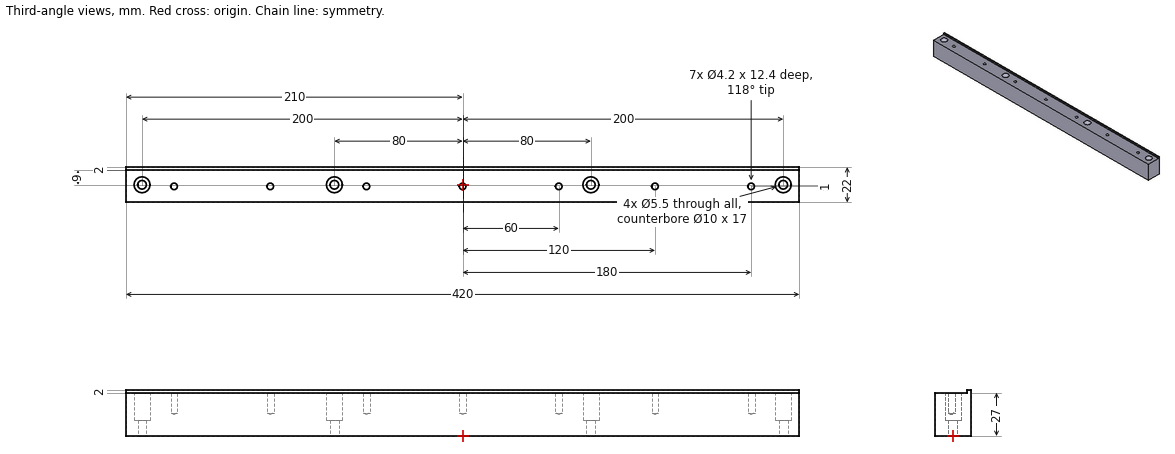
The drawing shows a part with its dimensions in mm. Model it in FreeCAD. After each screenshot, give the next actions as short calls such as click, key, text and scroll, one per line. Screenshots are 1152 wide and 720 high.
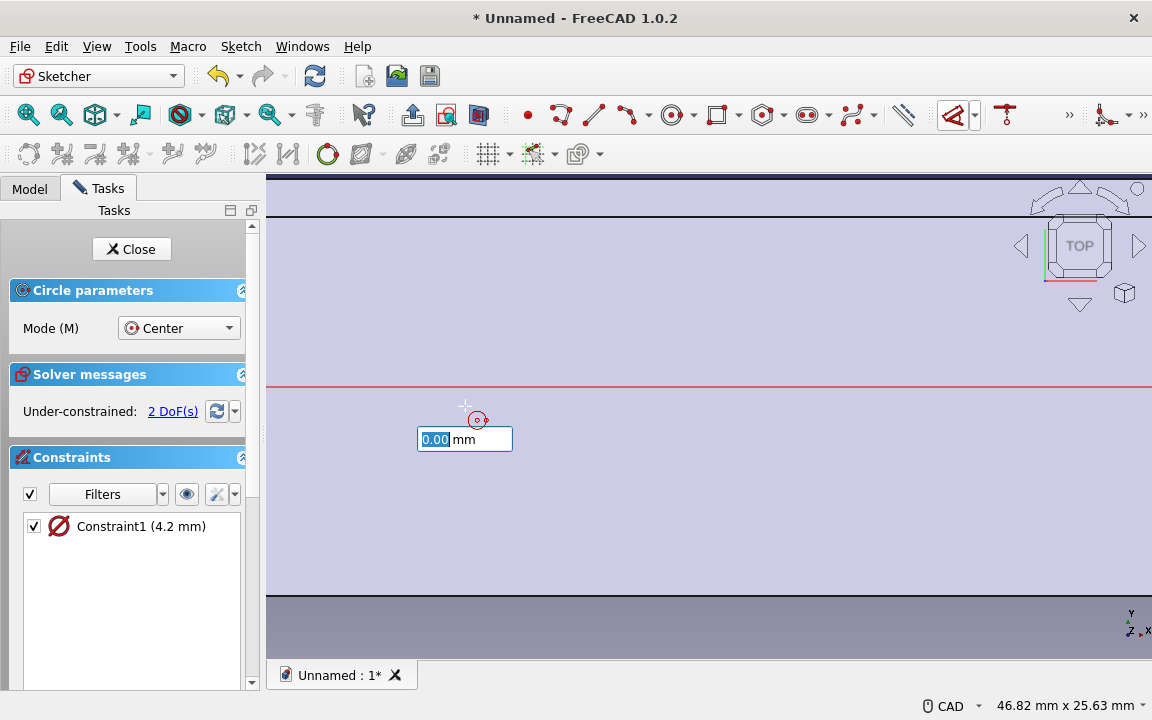
scroll(837, 417, down, 13)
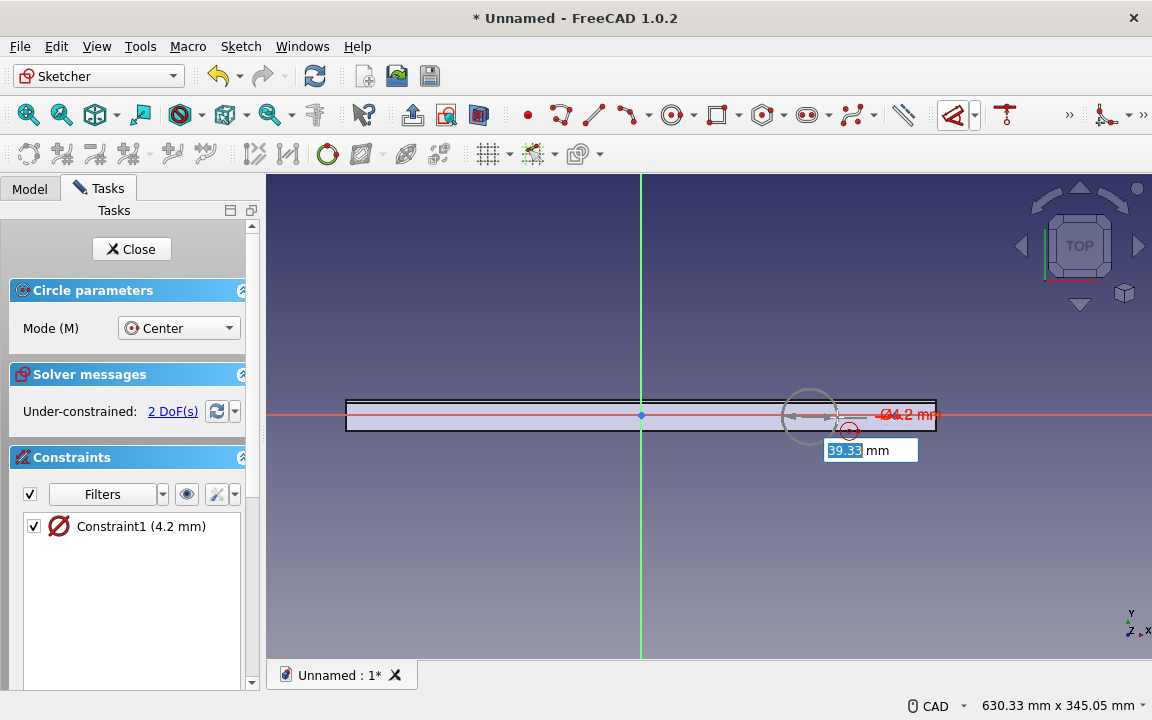
scroll(812, 419, up, 8)
move(810, 416)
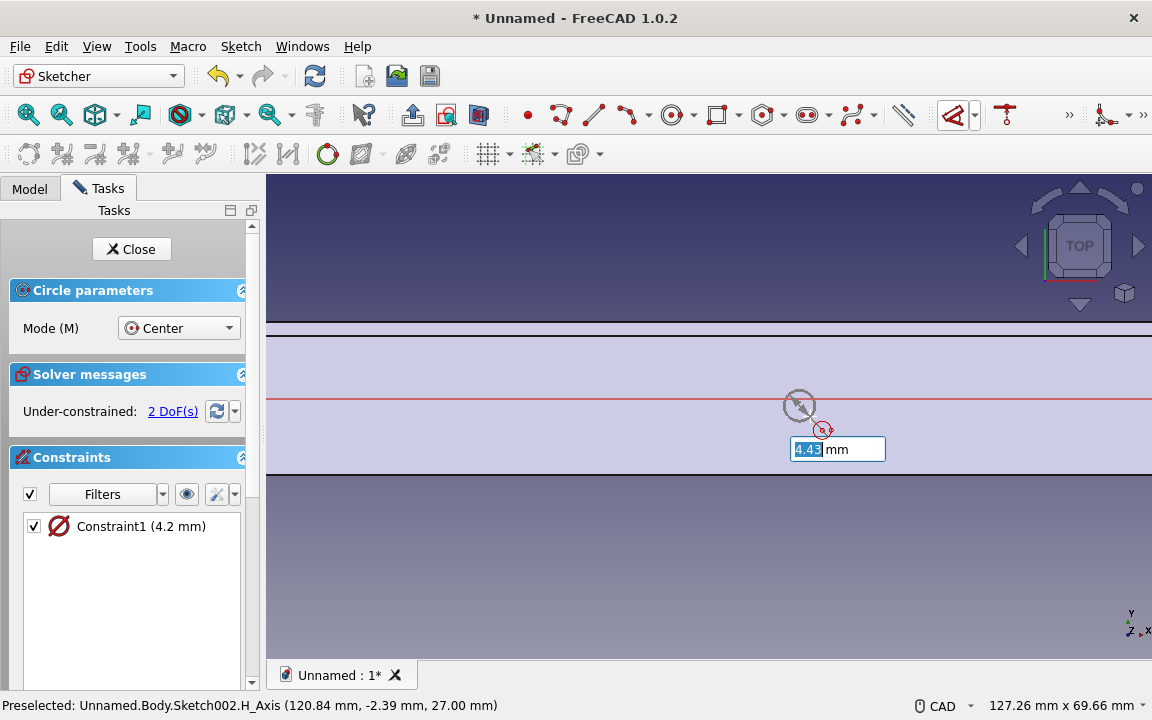
text(4.2)
key(Return)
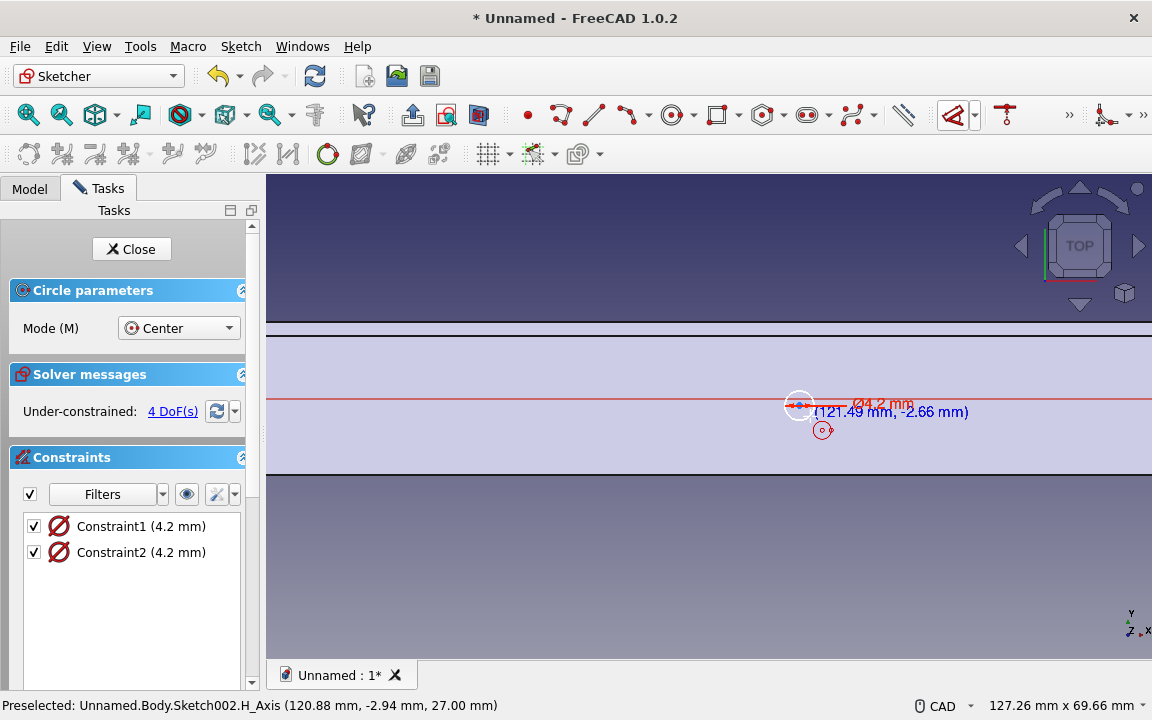
scroll(382, 405, up, 5)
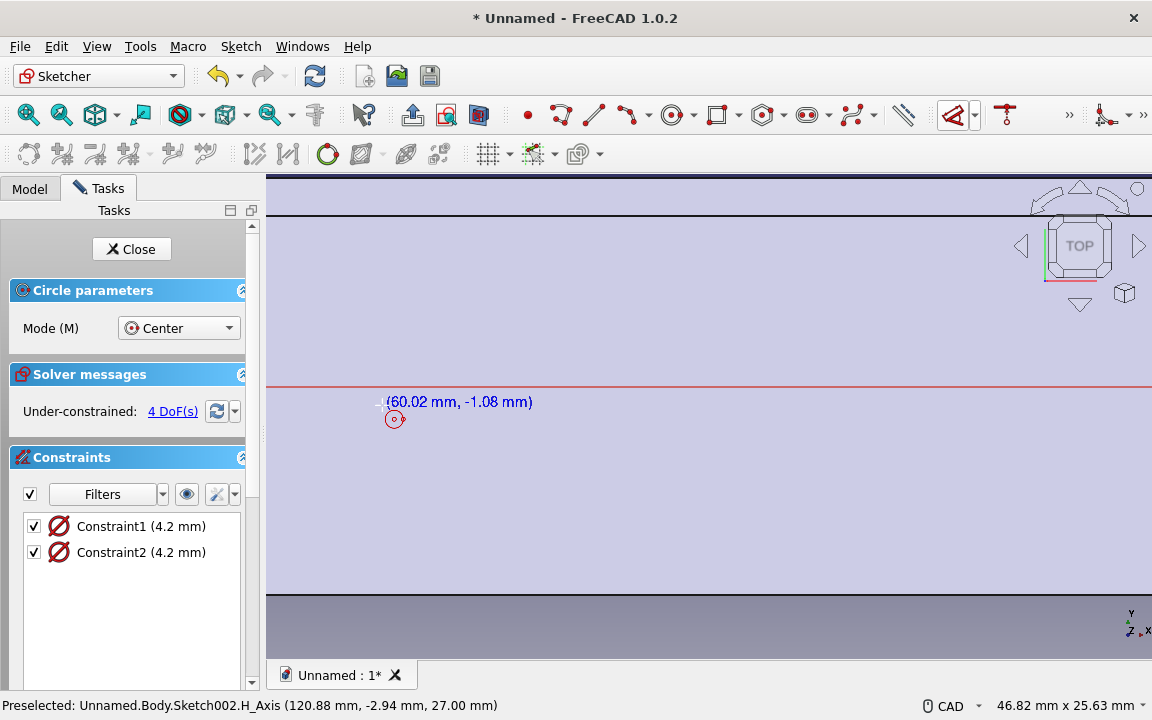
click(381, 405)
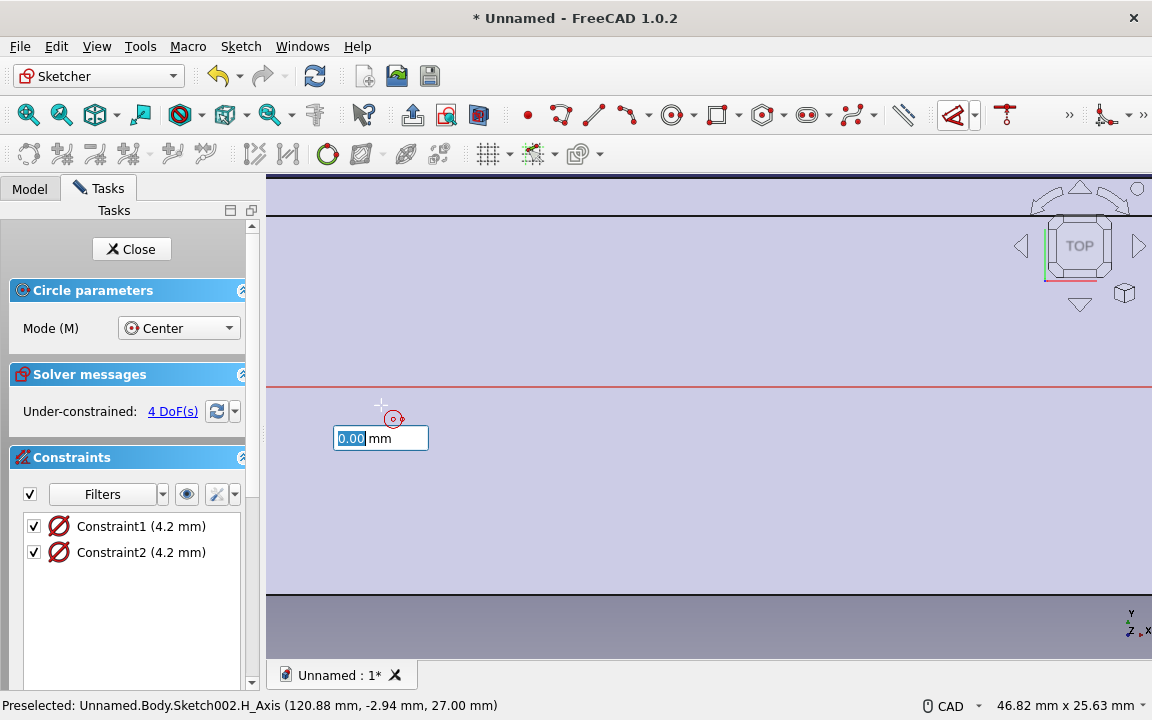
scroll(752, 417, down, 13)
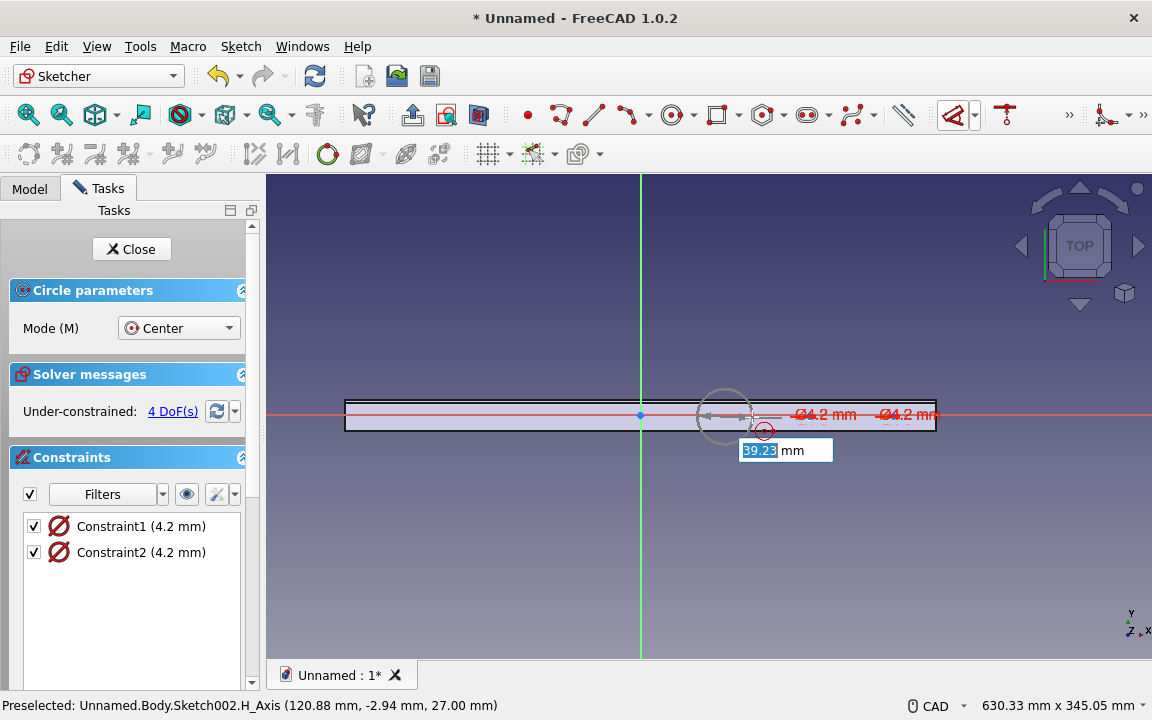
scroll(727, 419, up, 8)
move(725, 415)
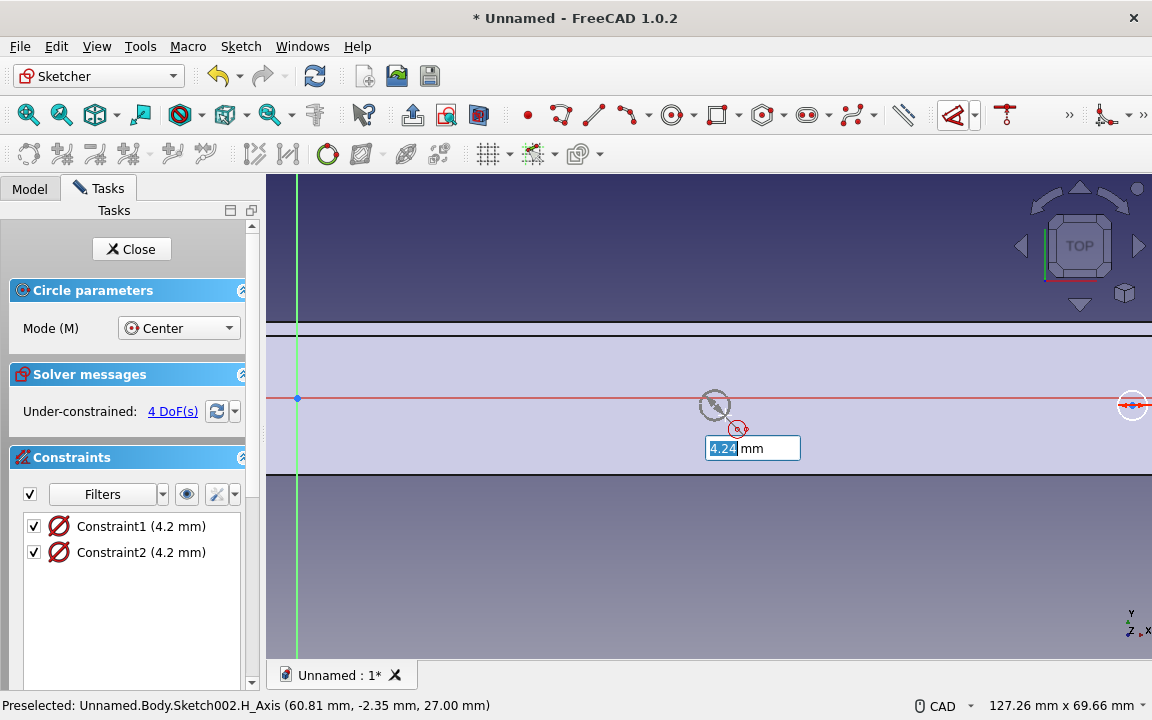
text(4.2)
key(Return)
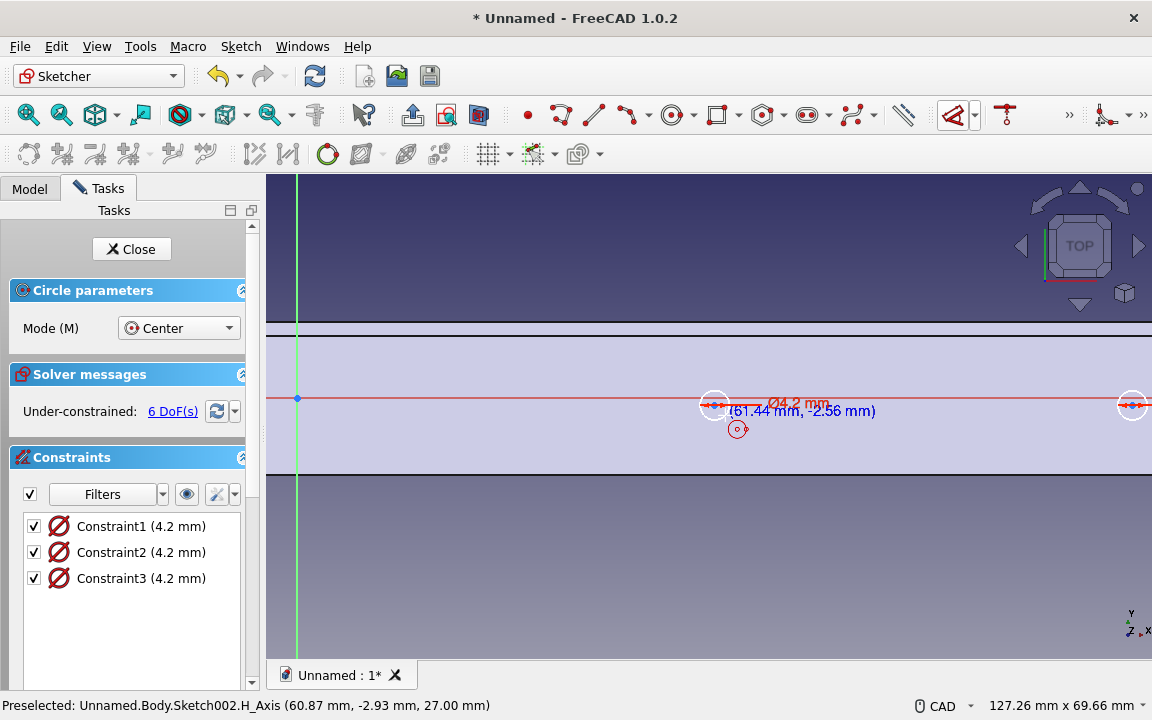
scroll(297, 405, up, 5)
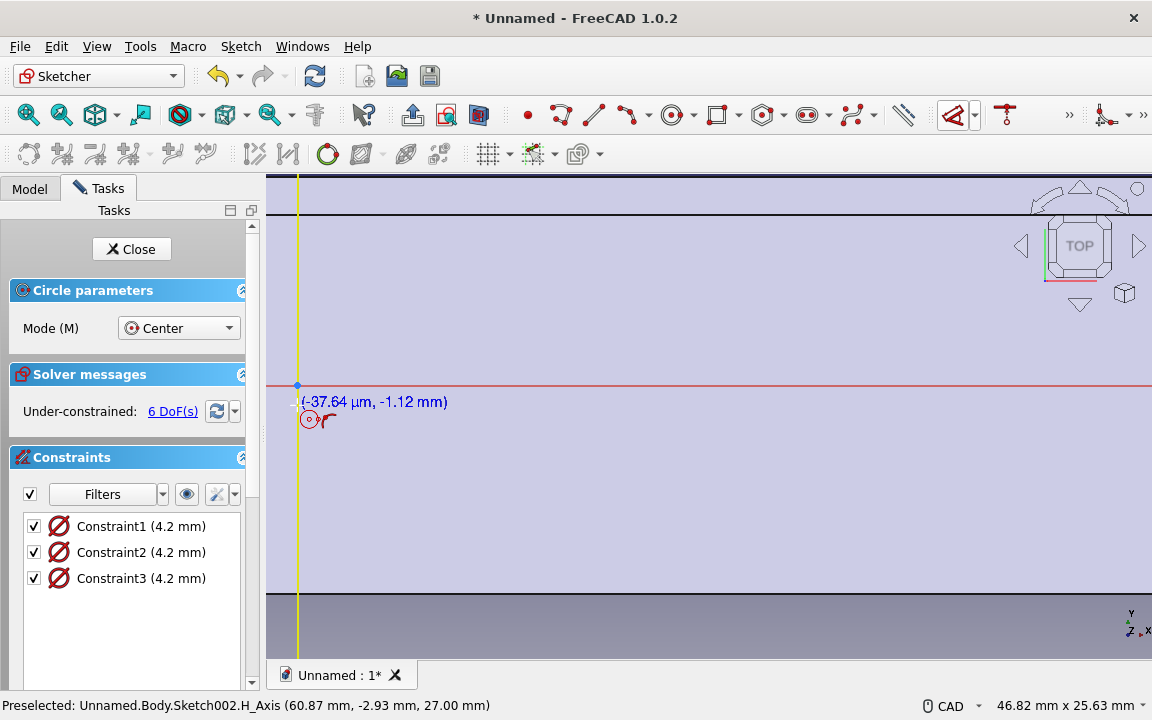
click(298, 405)
move(326, 433)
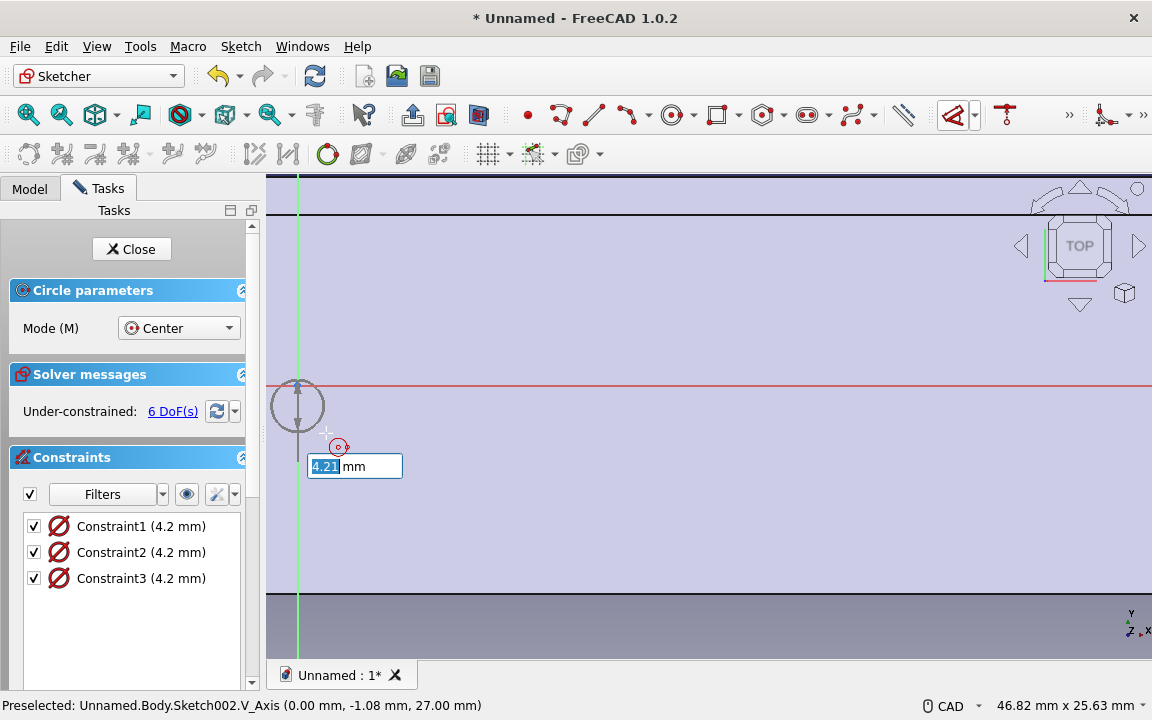
text(4.2)
key(Return)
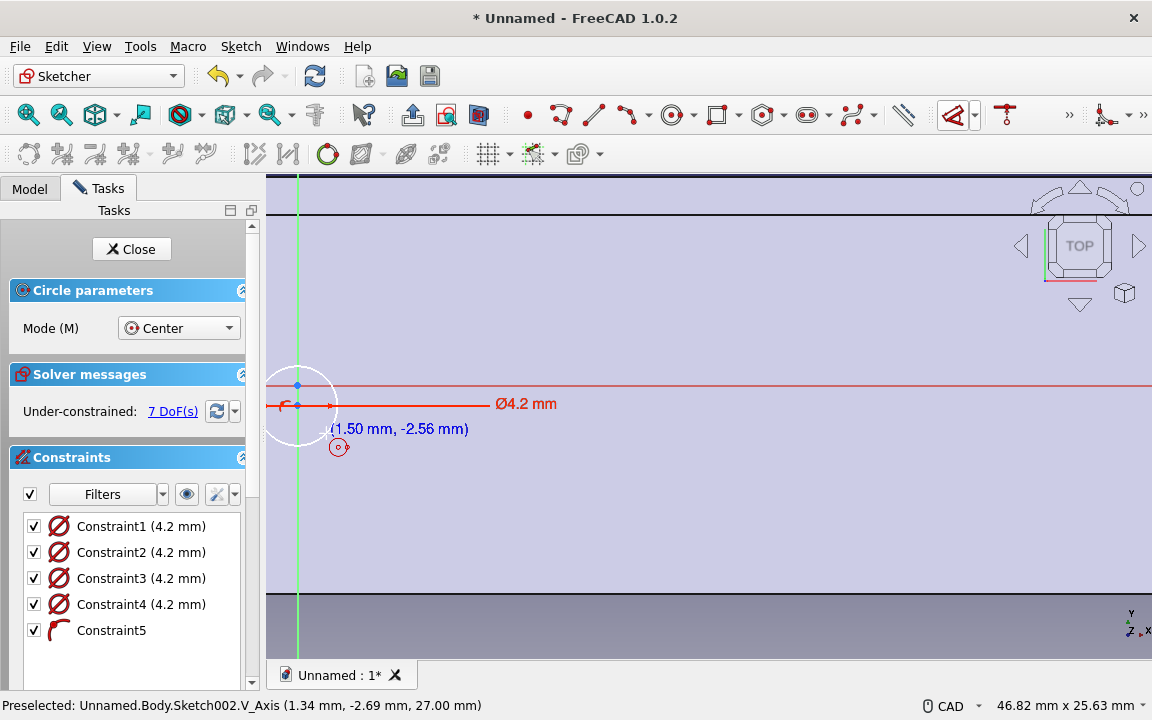
scroll(668, 417, down, 13)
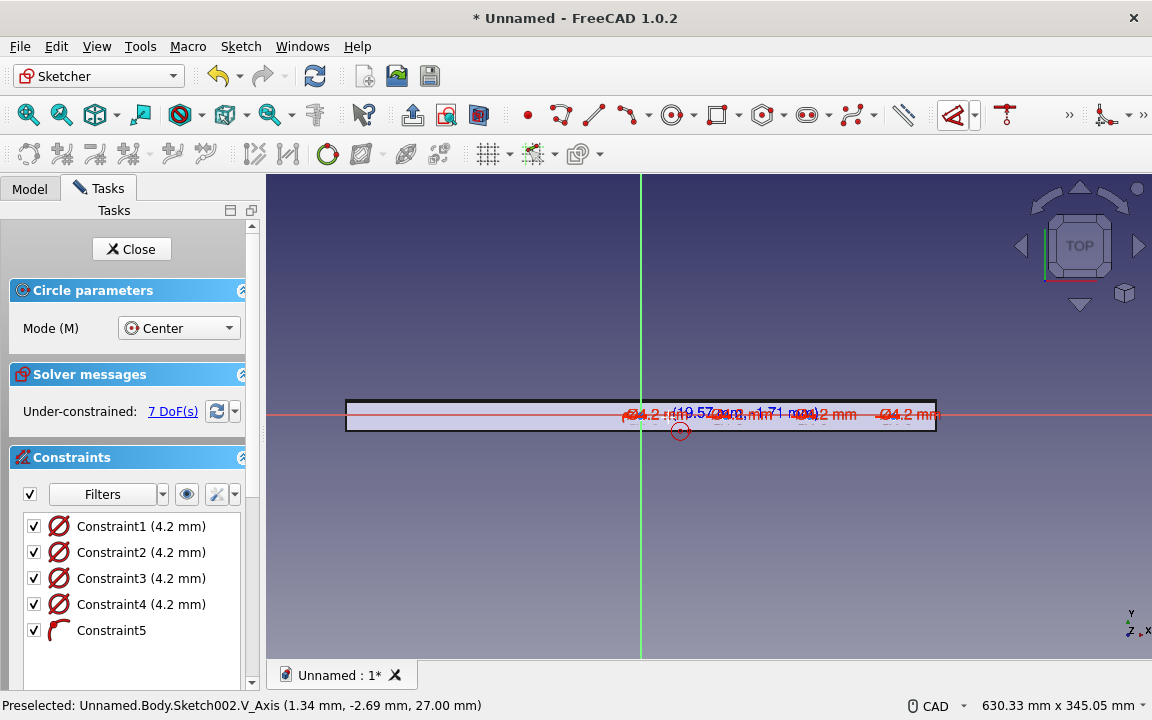
scroll(388, 417, up, 13)